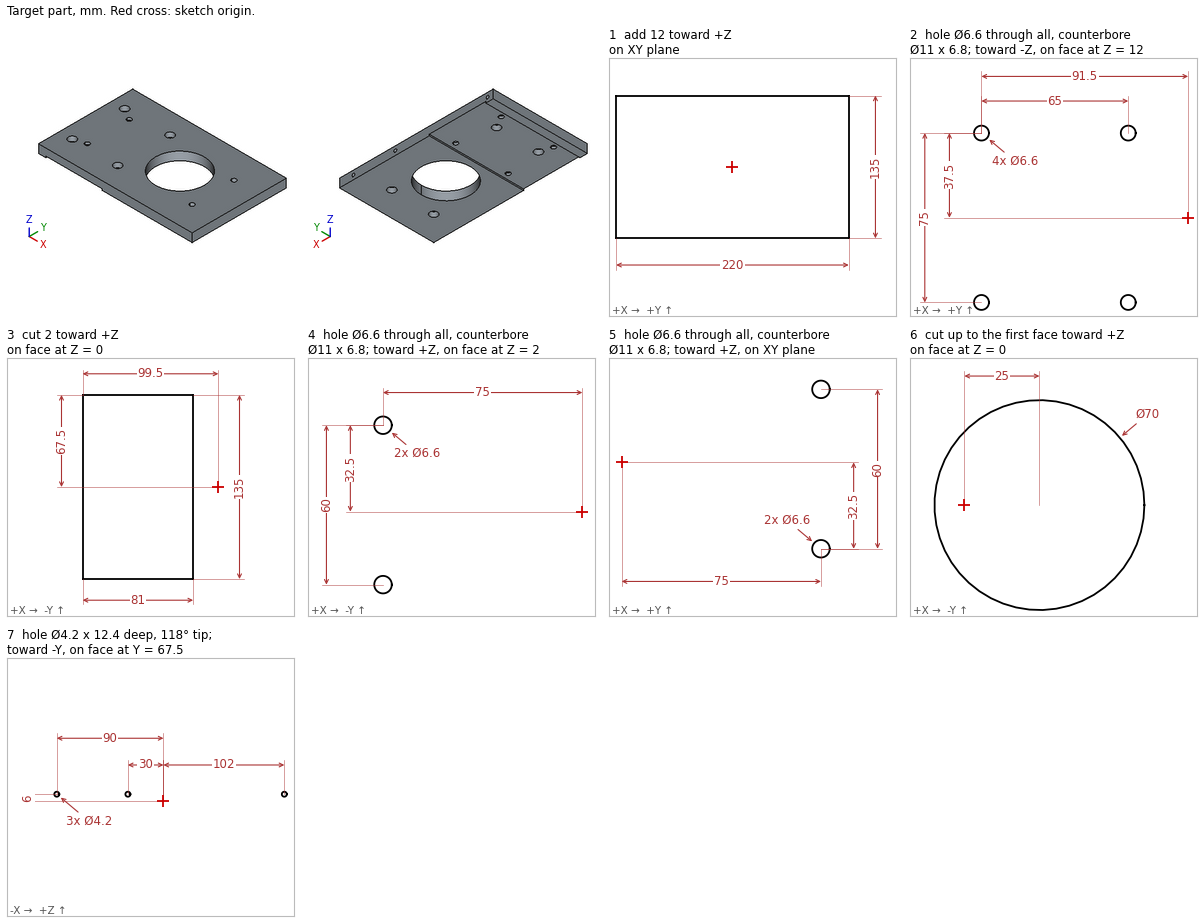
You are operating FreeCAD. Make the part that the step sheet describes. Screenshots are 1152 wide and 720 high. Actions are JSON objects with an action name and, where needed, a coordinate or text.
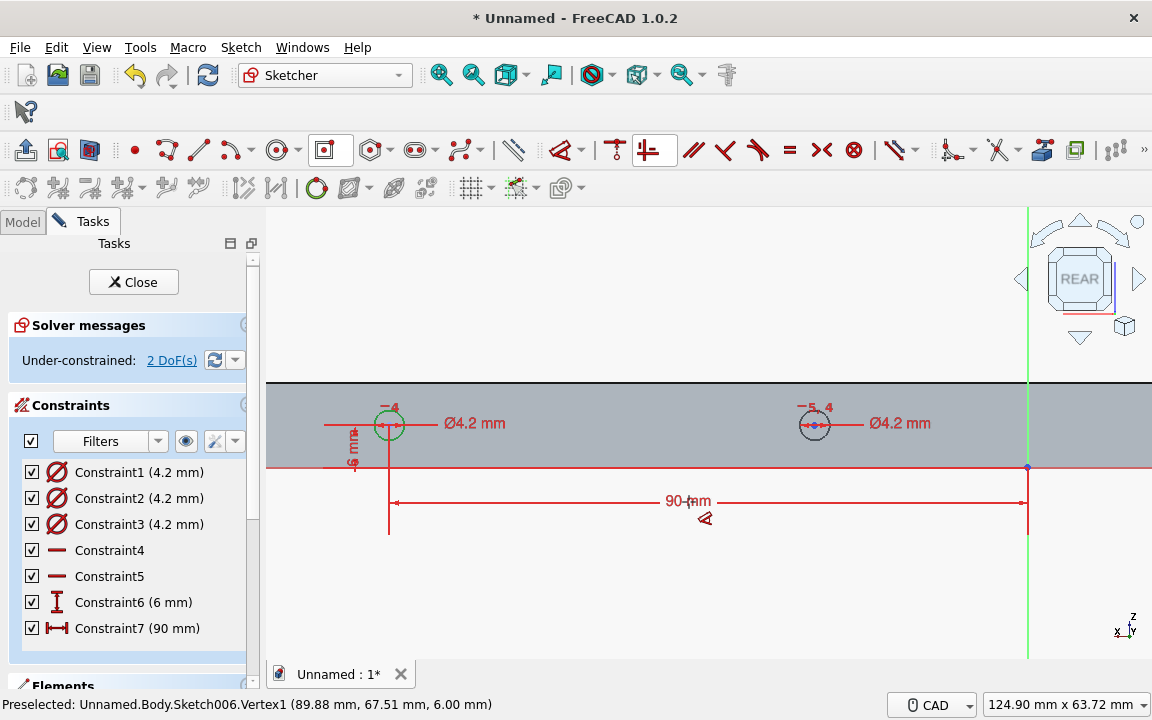
{"action": "left_click", "coordinate": [815, 425]}
{"action": "left_click", "coordinate": [901, 502]}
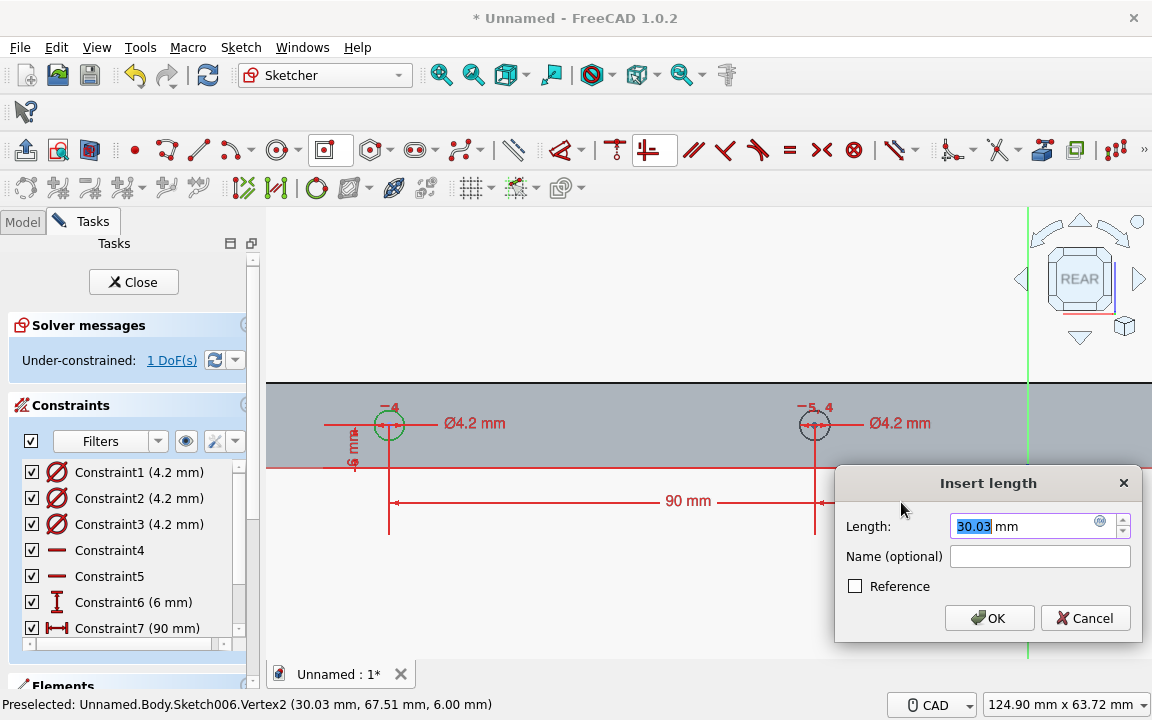
{"action": "type", "text": "30"}
{"action": "key", "text": "Return"}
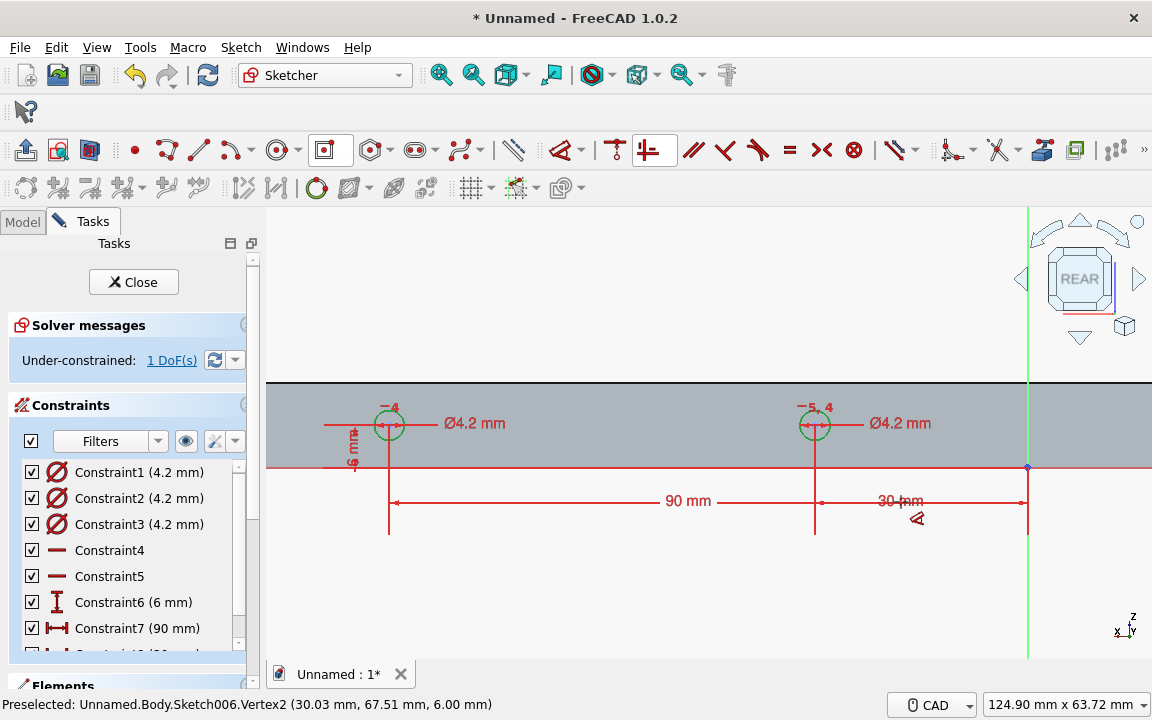
{"action": "scroll", "coordinate": [390, 429], "scroll_direction": "down", "scroll_amount": 5}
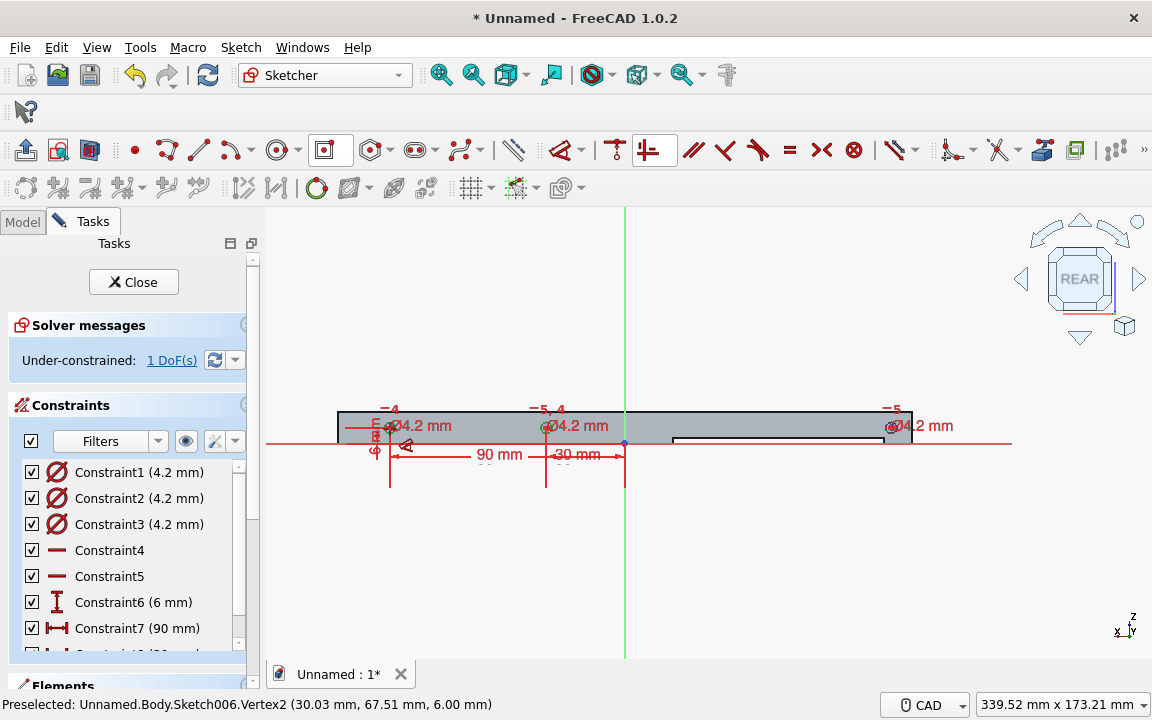
{"action": "left_click", "coordinate": [891, 428]}
{"action": "left_click", "coordinate": [758, 478]}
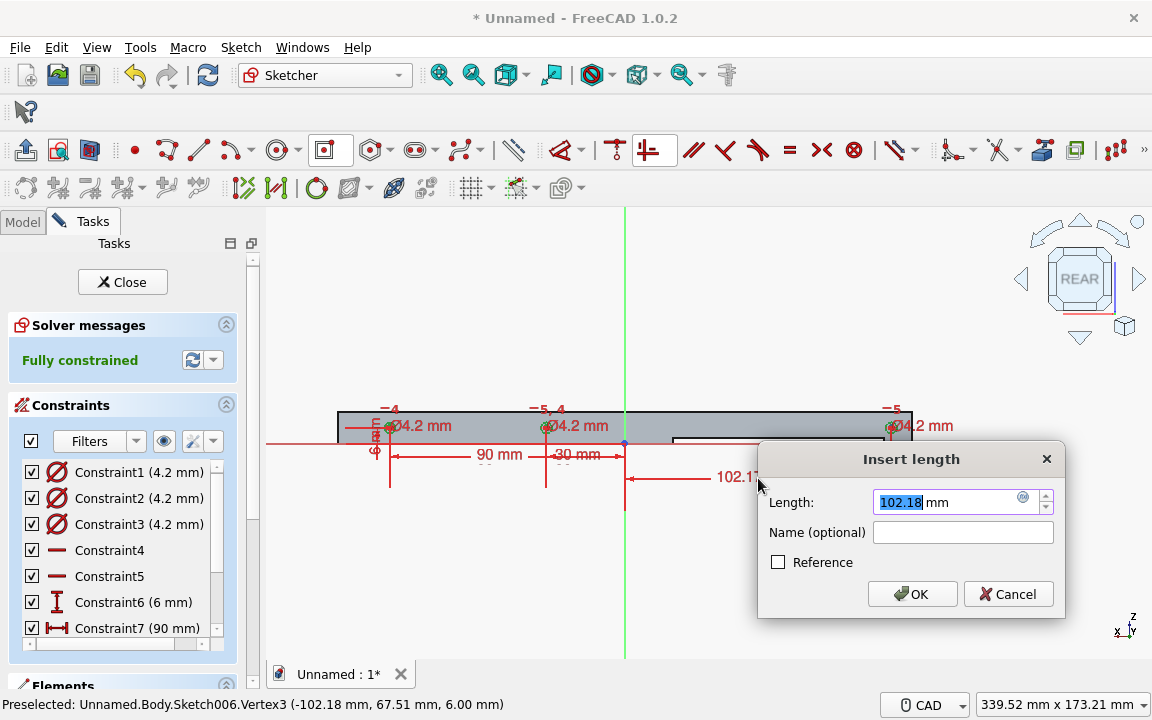
{"action": "type", "text": "102"}
{"action": "key", "text": "Return"}
{"action": "key", "text": "Escape"}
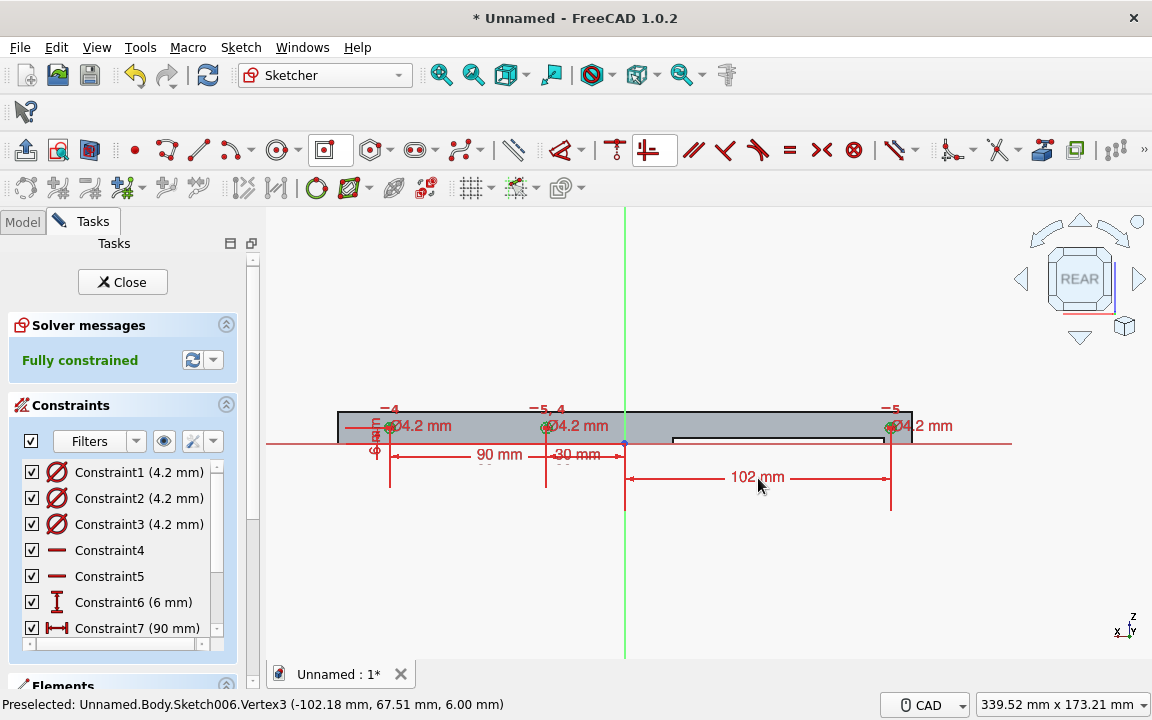
{"action": "left_click", "coordinate": [123, 282]}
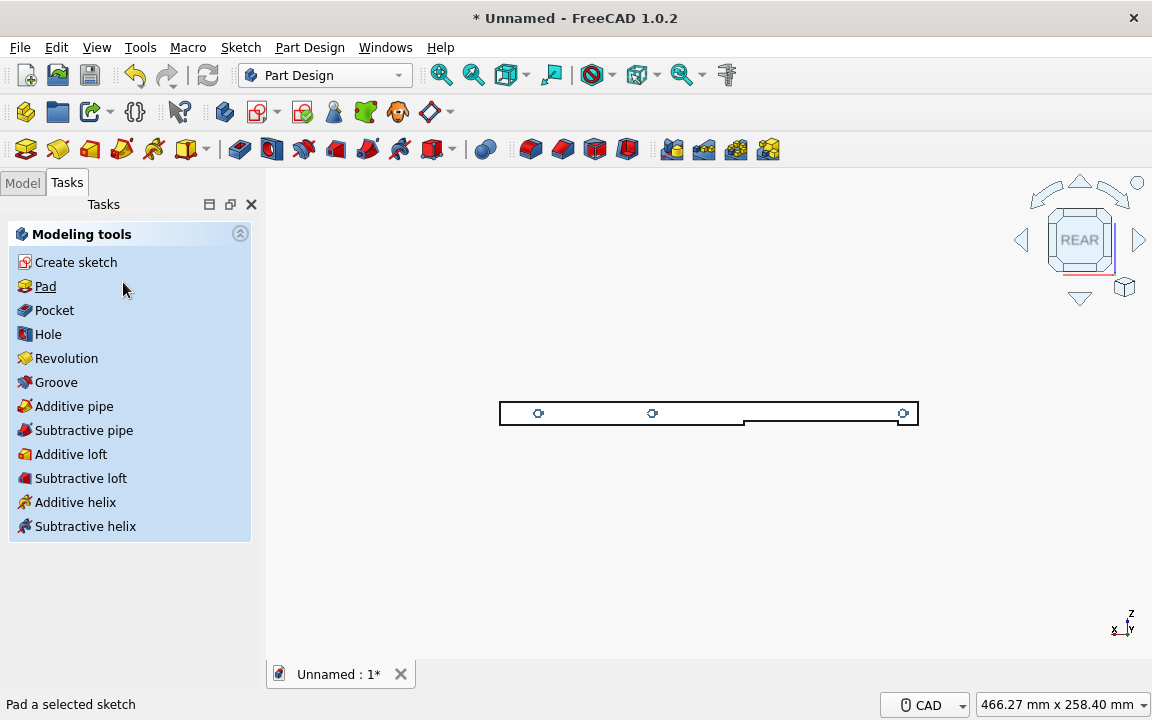
{"action": "left_click", "coordinate": [272, 150]}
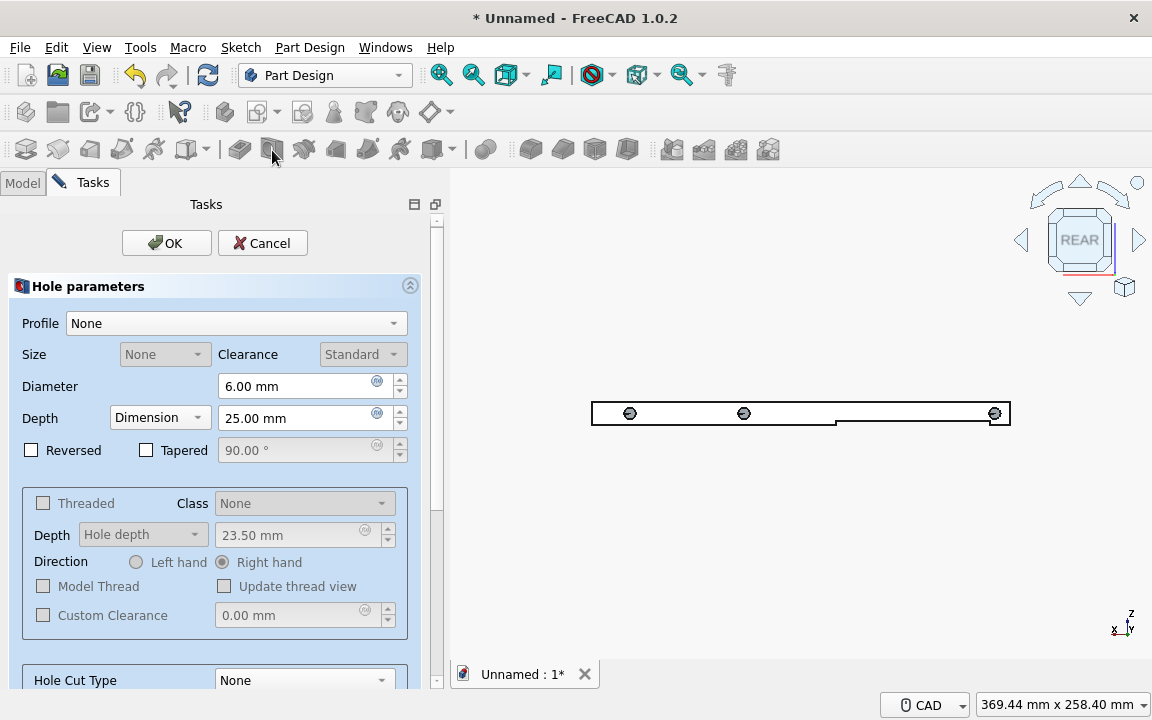
{"action": "triple_click", "coordinate": [305, 386]}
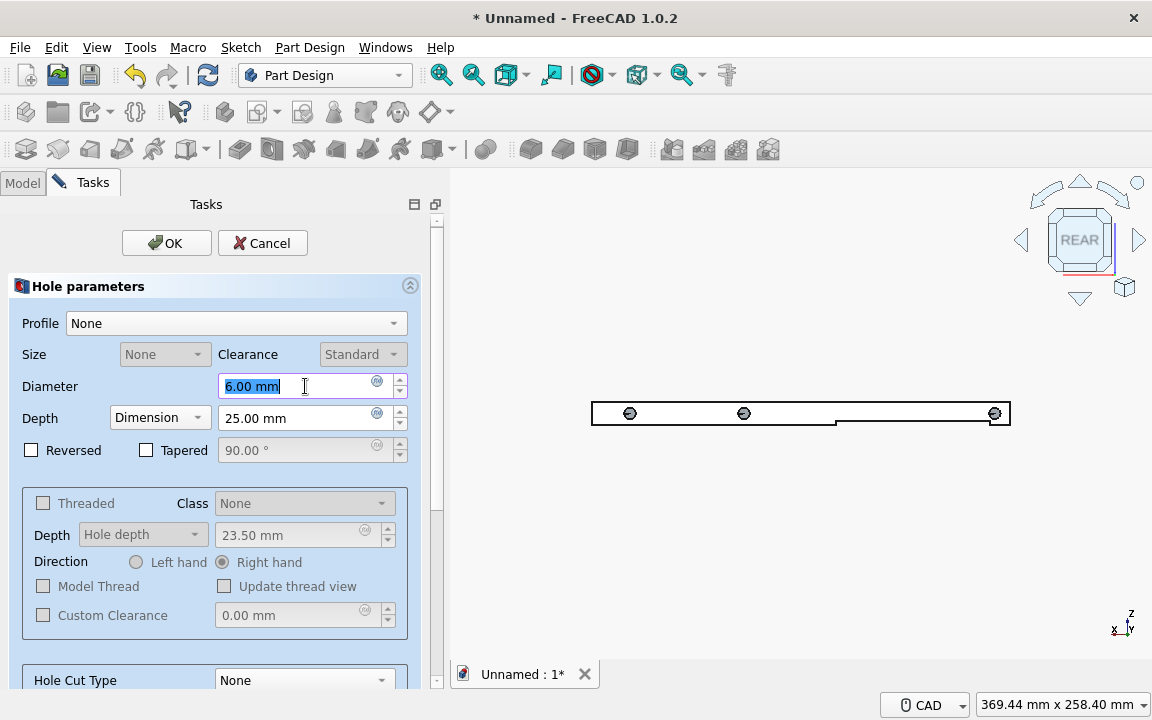
{"action": "type", "text": "4.2"}
{"action": "key", "text": "Tab"}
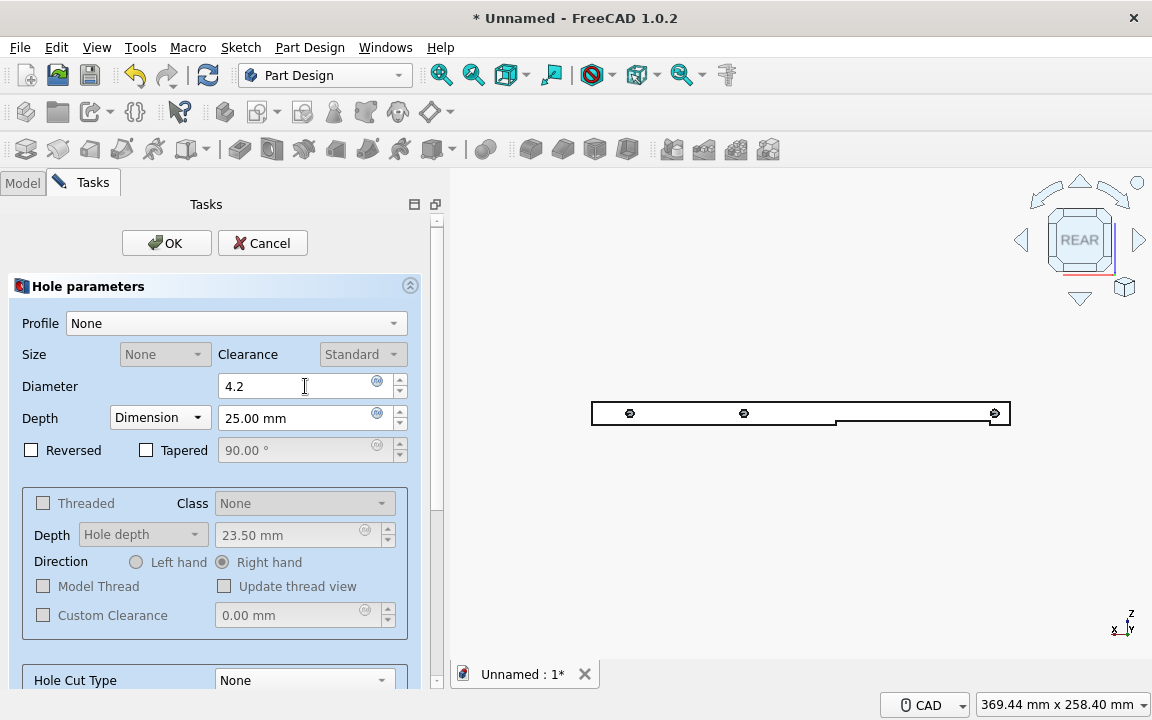
{"action": "triple_click", "coordinate": [305, 418]}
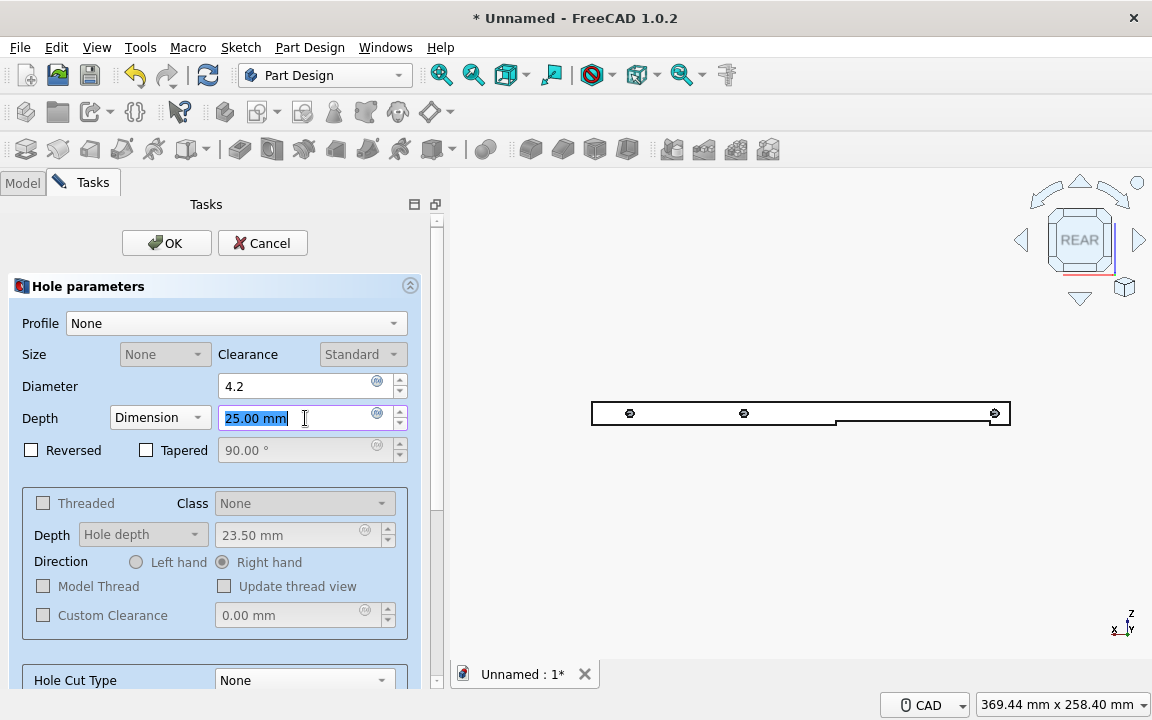
{"action": "type", "text": "12.4"}
{"action": "key", "text": "Tab"}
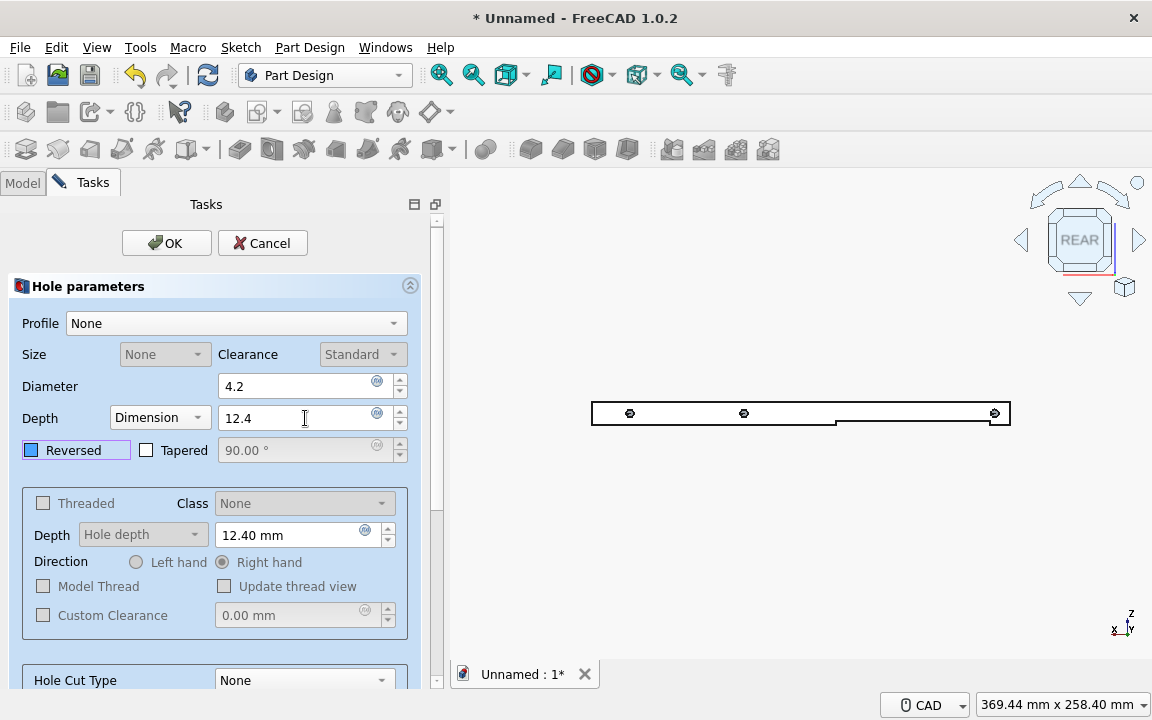
{"action": "left_click", "coordinate": [167, 243]}